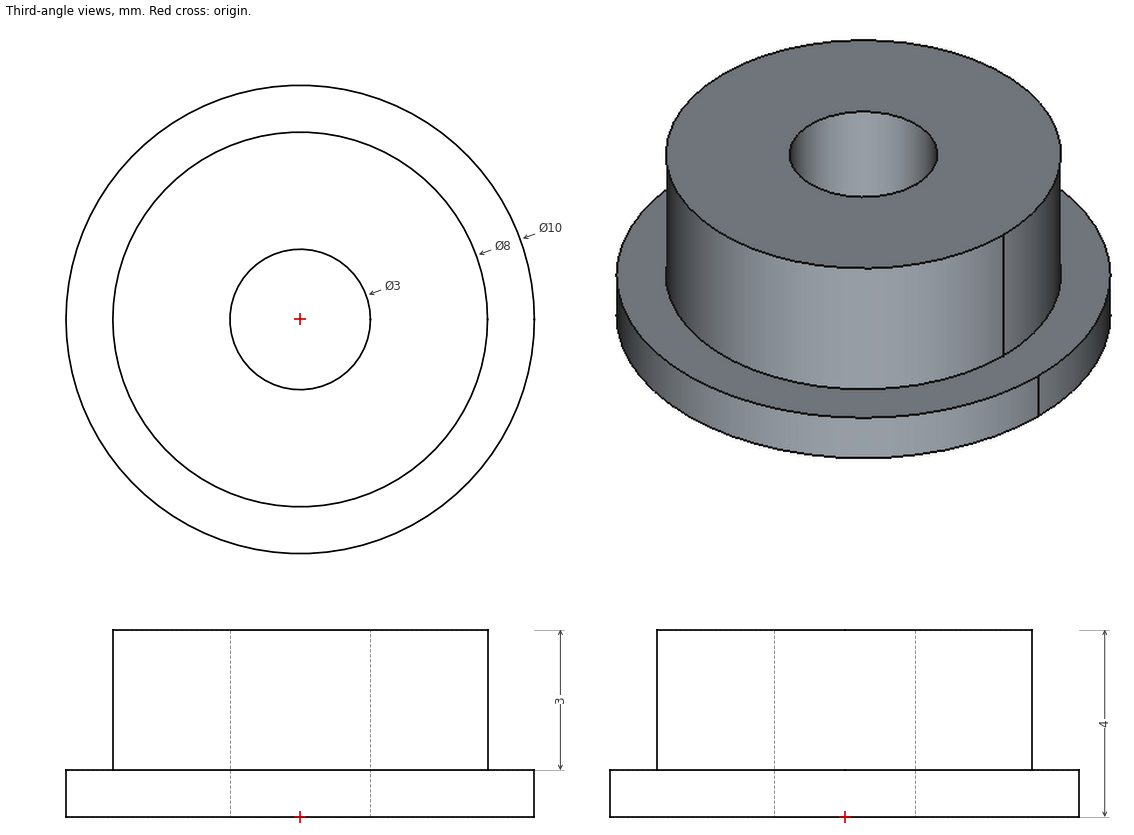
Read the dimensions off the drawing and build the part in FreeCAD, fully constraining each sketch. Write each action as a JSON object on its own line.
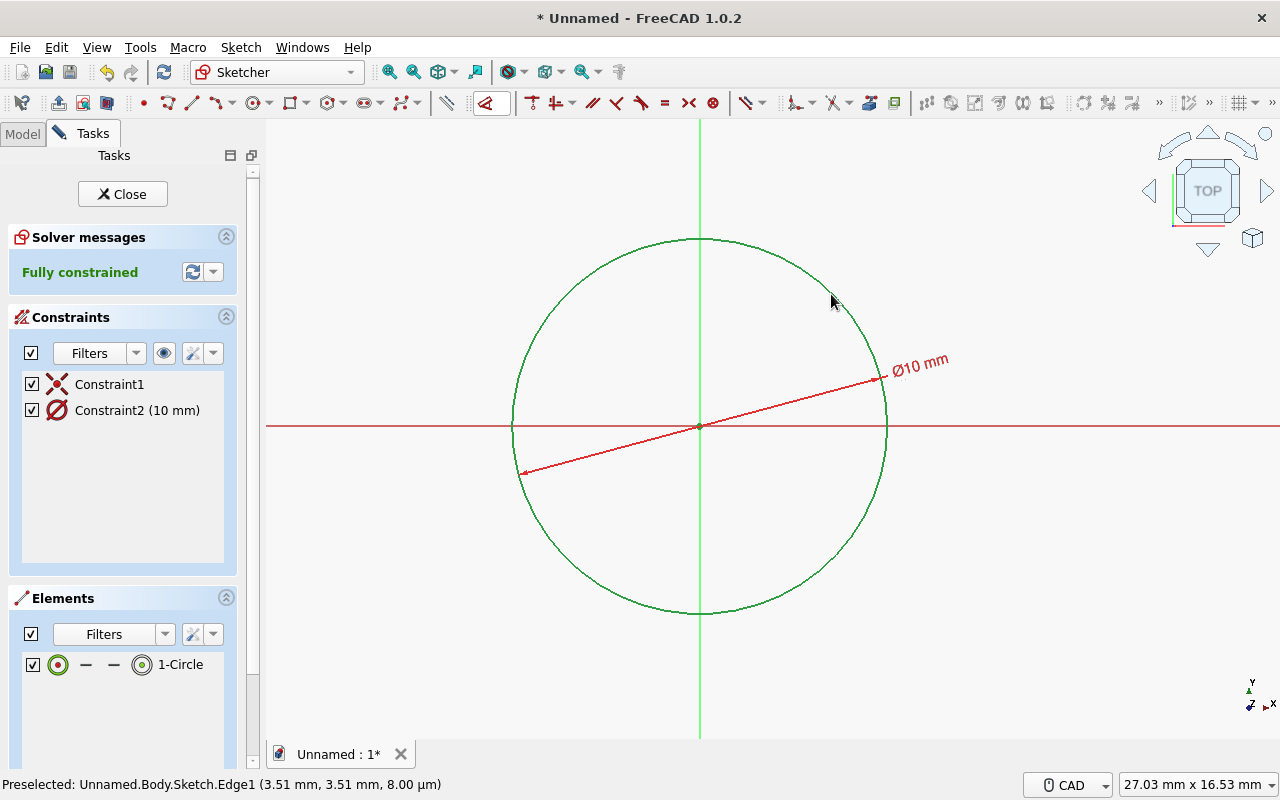
{"action": "left_click", "coordinate": [123, 194]}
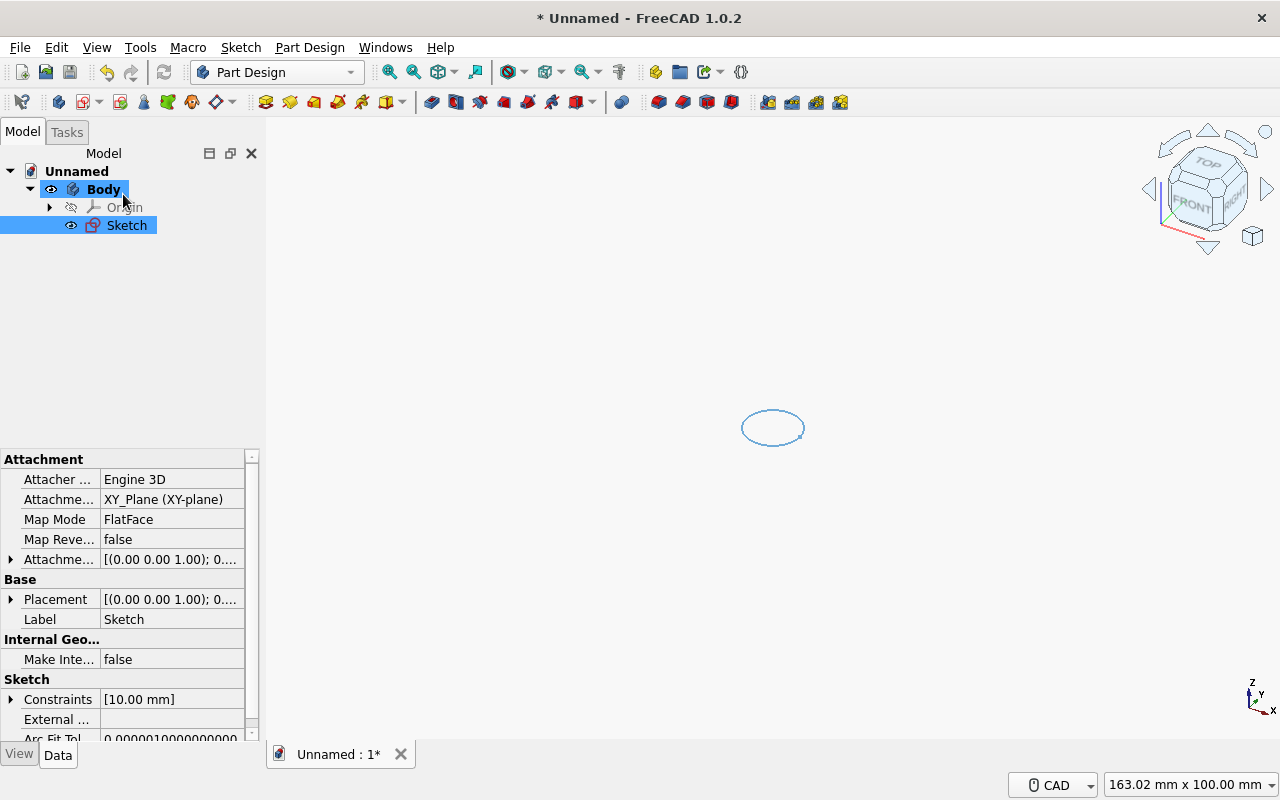
{"action": "left_click", "coordinate": [266, 102]}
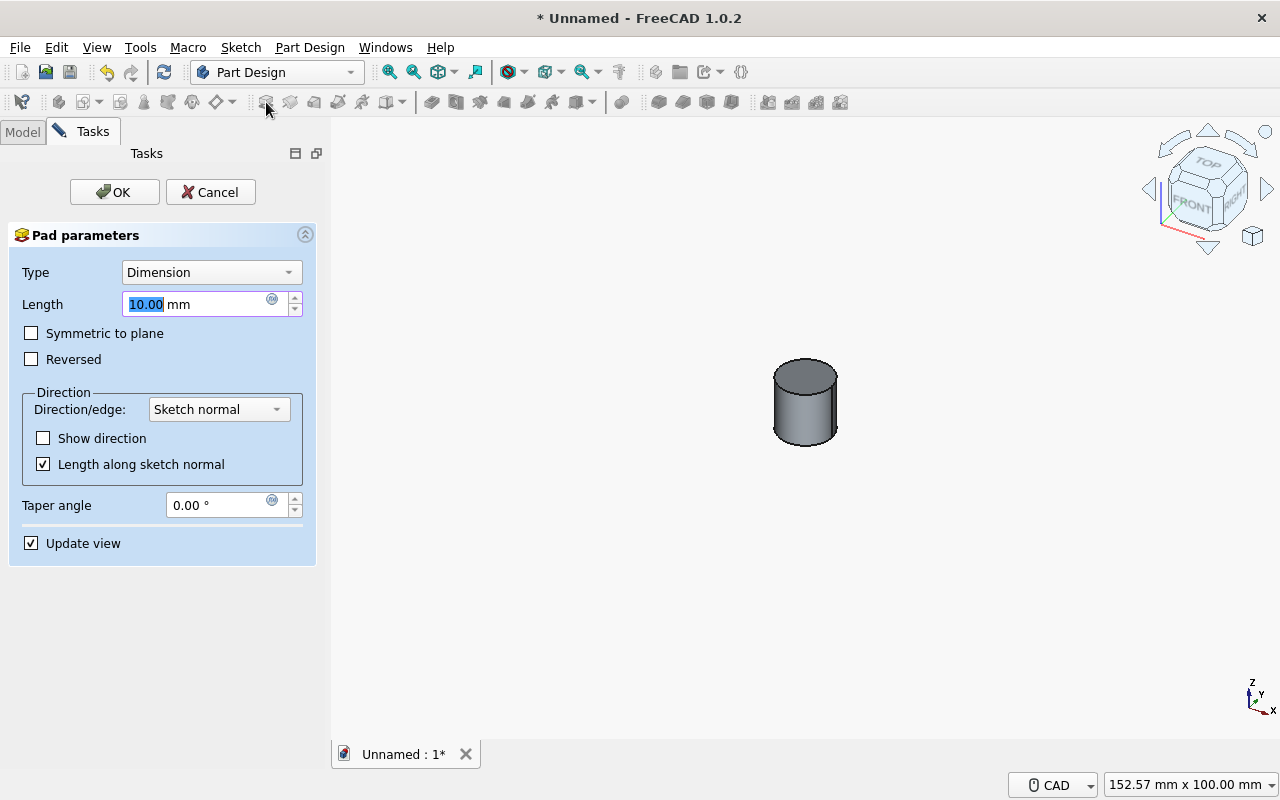
{"action": "type", "text": "4"}
{"action": "key", "text": "Tab"}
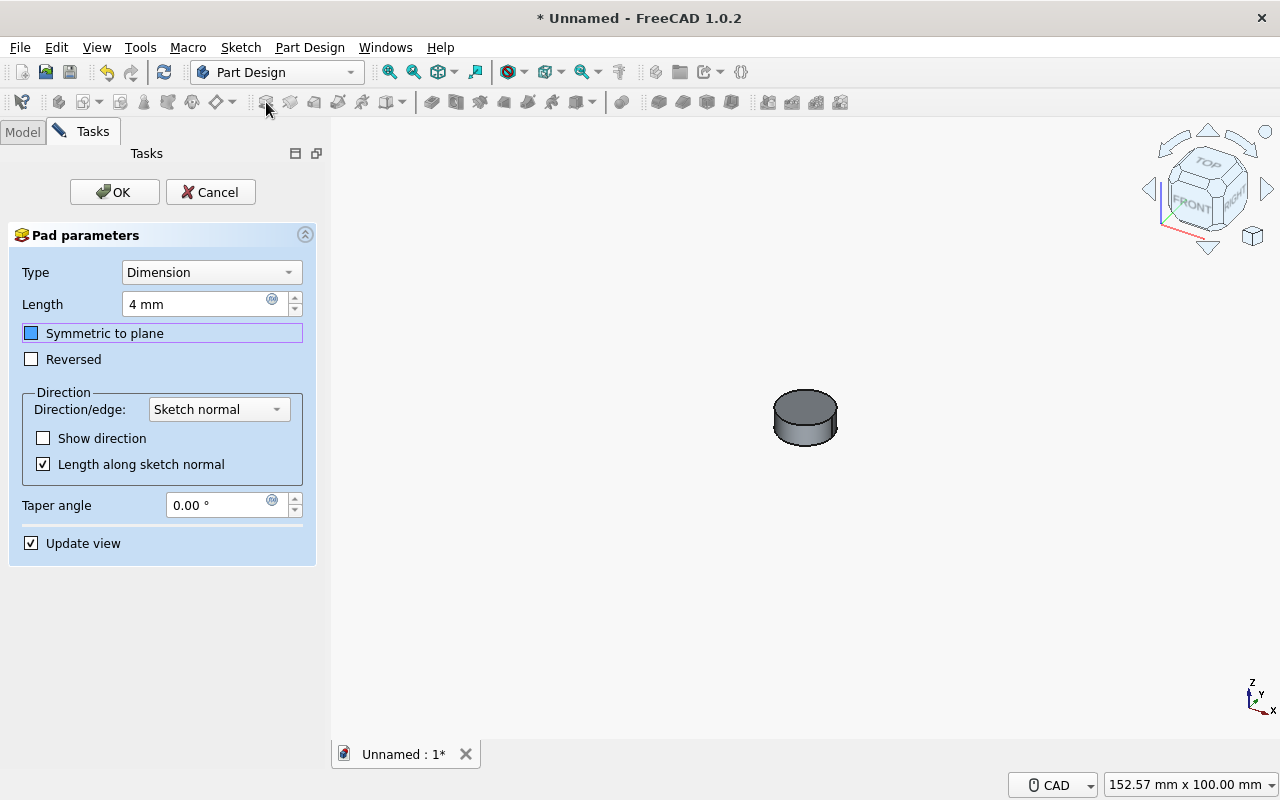
{"action": "left_click", "coordinate": [115, 192]}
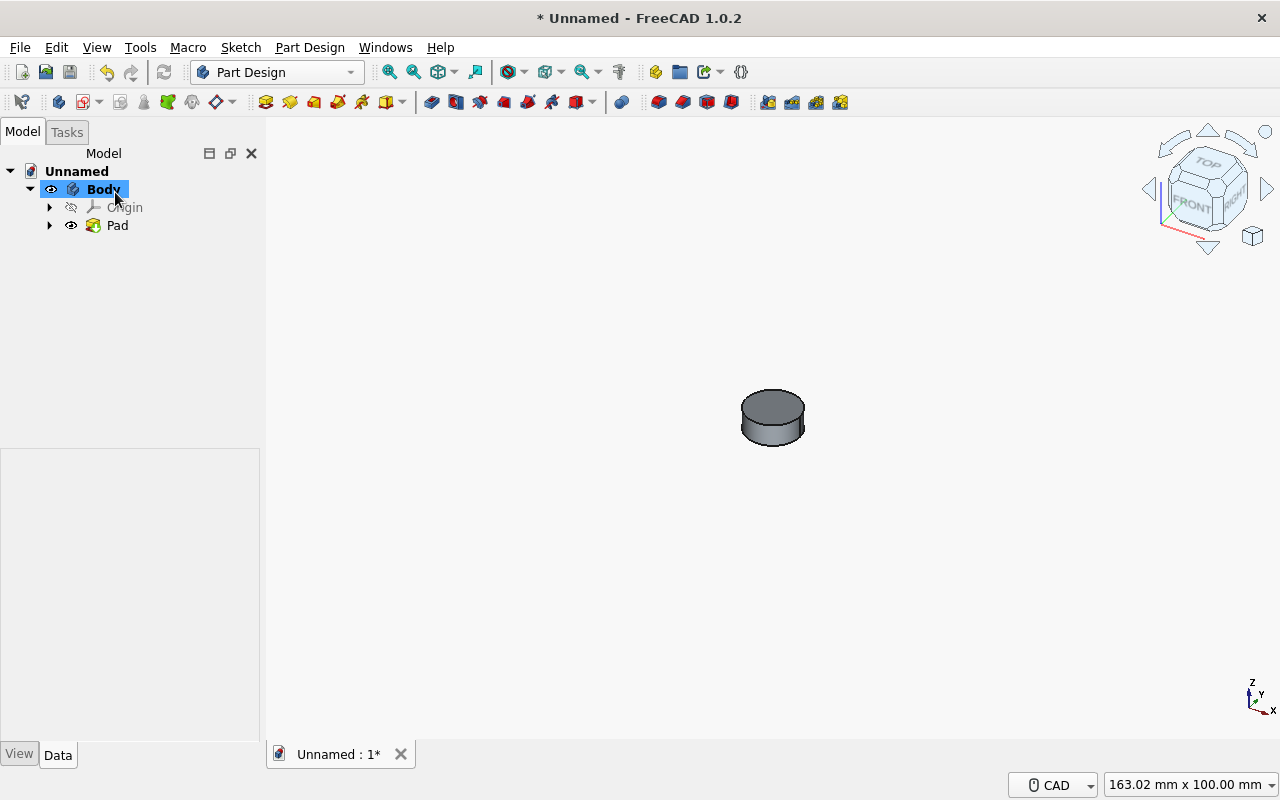
{"action": "left_click", "coordinate": [390, 72]}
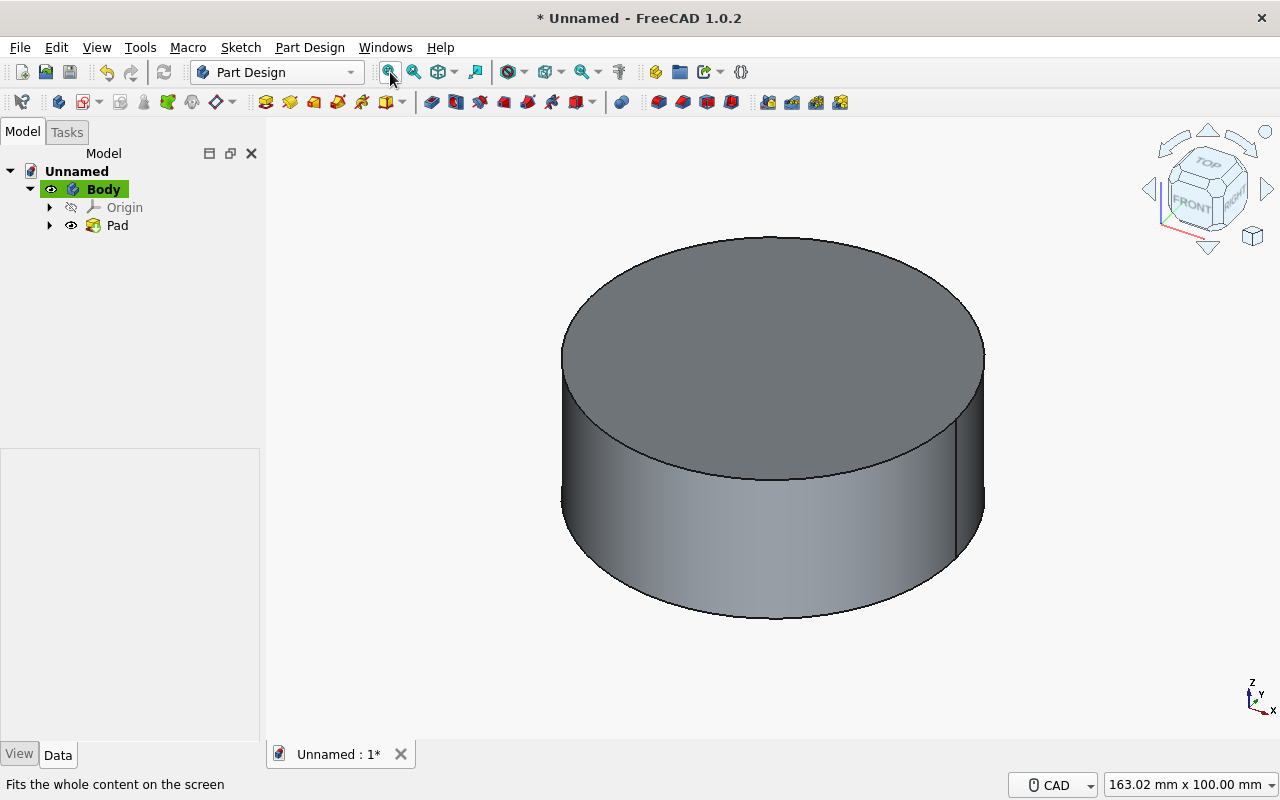
{"action": "left_click", "coordinate": [50, 207]}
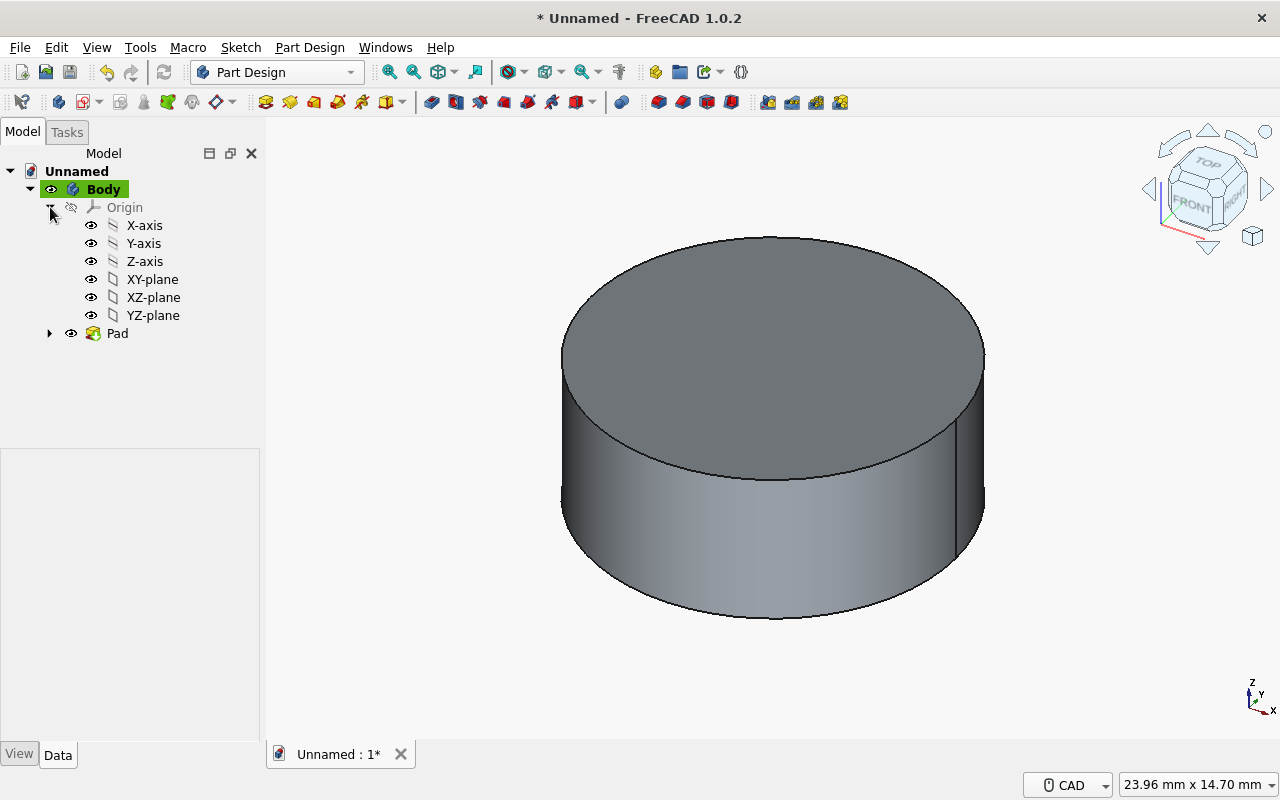
{"action": "left_click", "coordinate": [136, 279]}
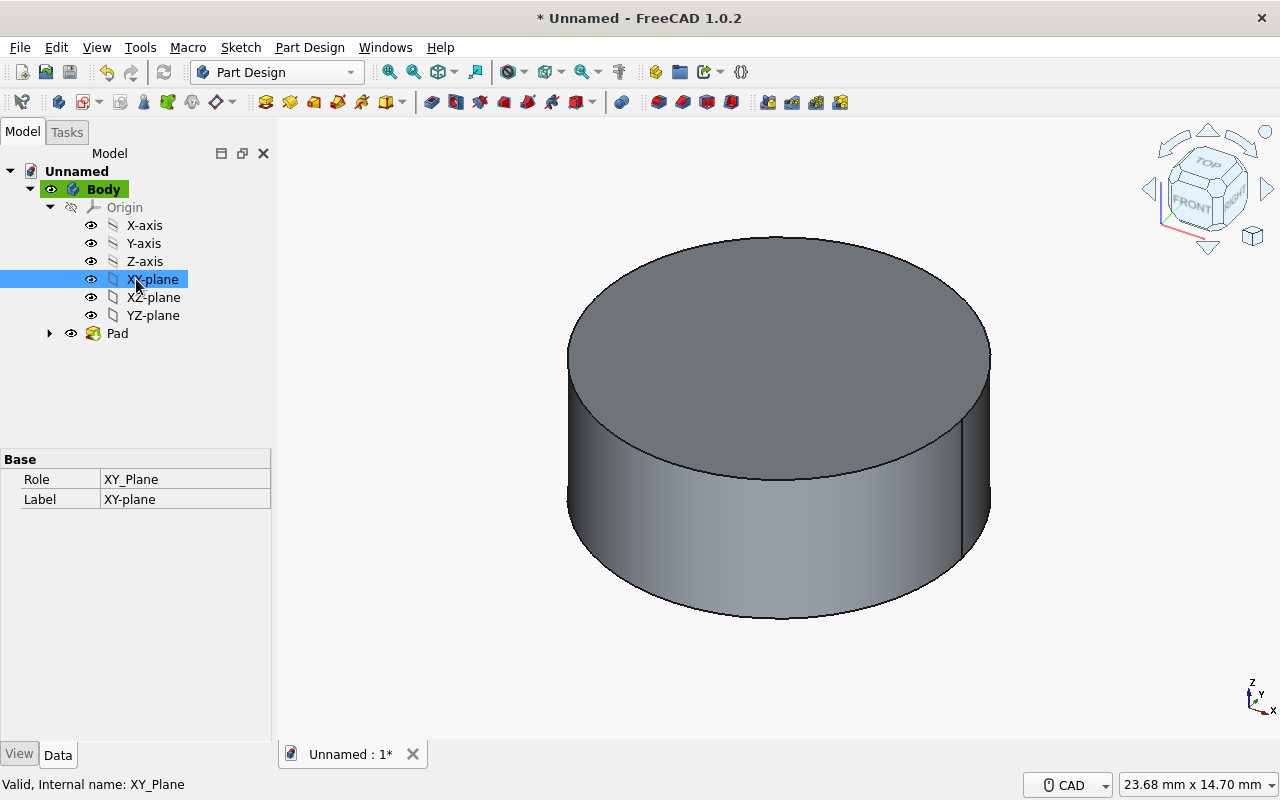
{"action": "left_click", "coordinate": [216, 102]}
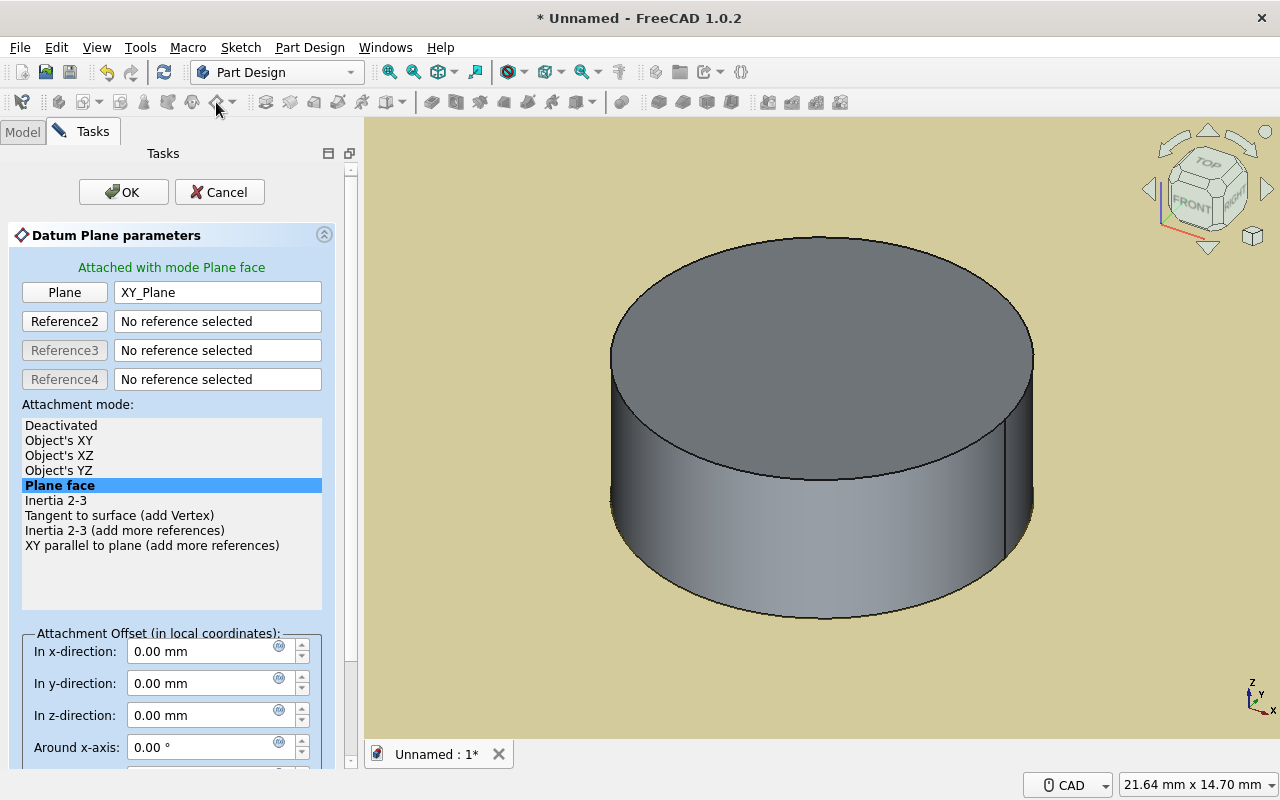
{"action": "triple_click", "coordinate": [210, 715]}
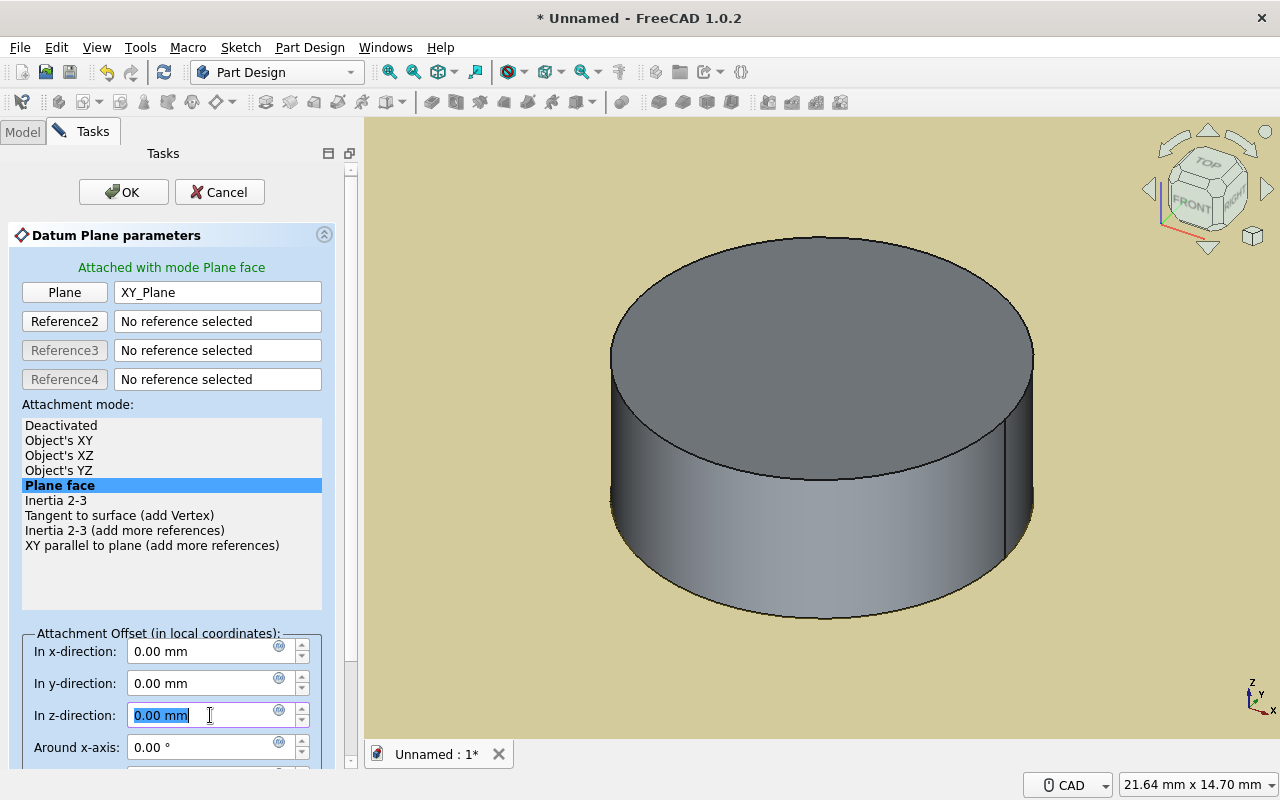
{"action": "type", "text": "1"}
{"action": "key", "text": "Tab"}